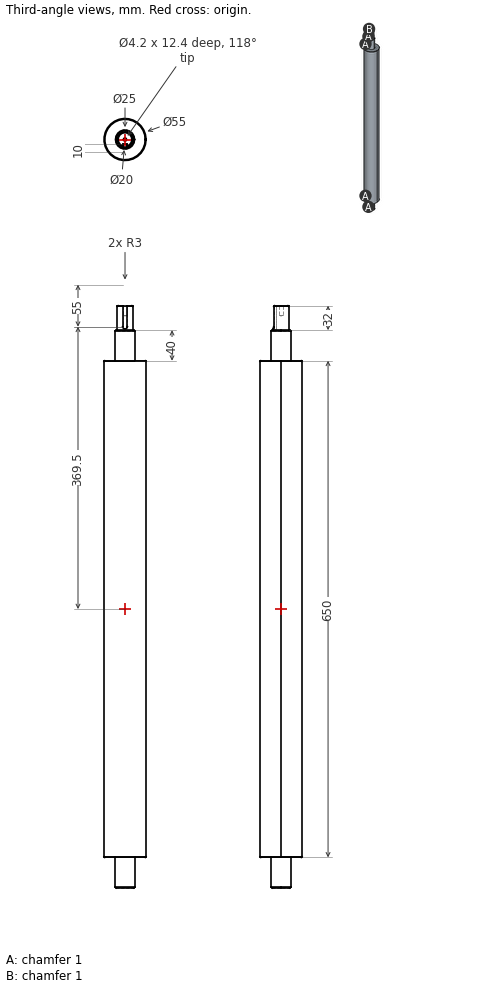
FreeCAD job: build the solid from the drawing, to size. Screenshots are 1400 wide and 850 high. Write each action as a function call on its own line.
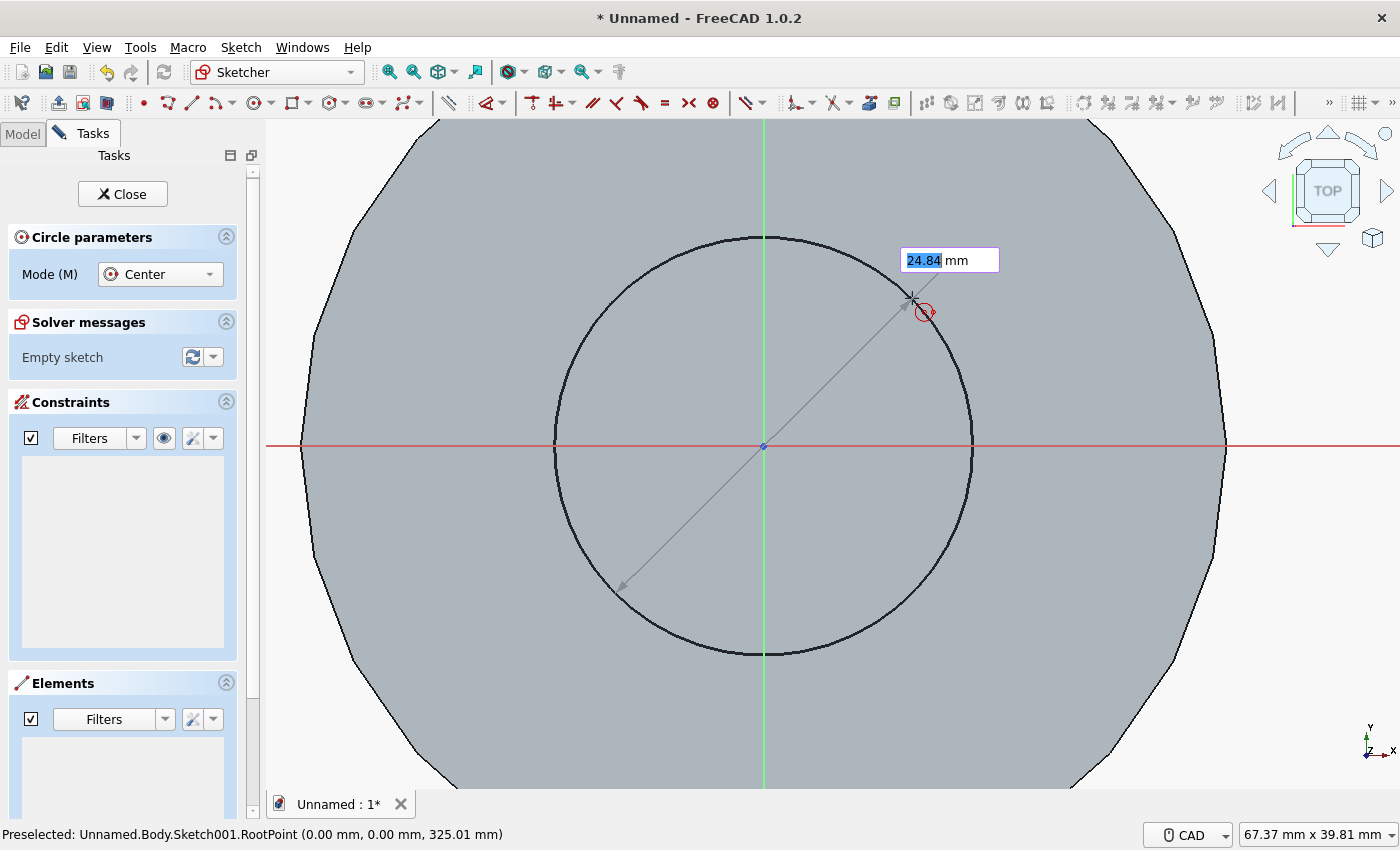
text(25)
key(Return)
key(Escape)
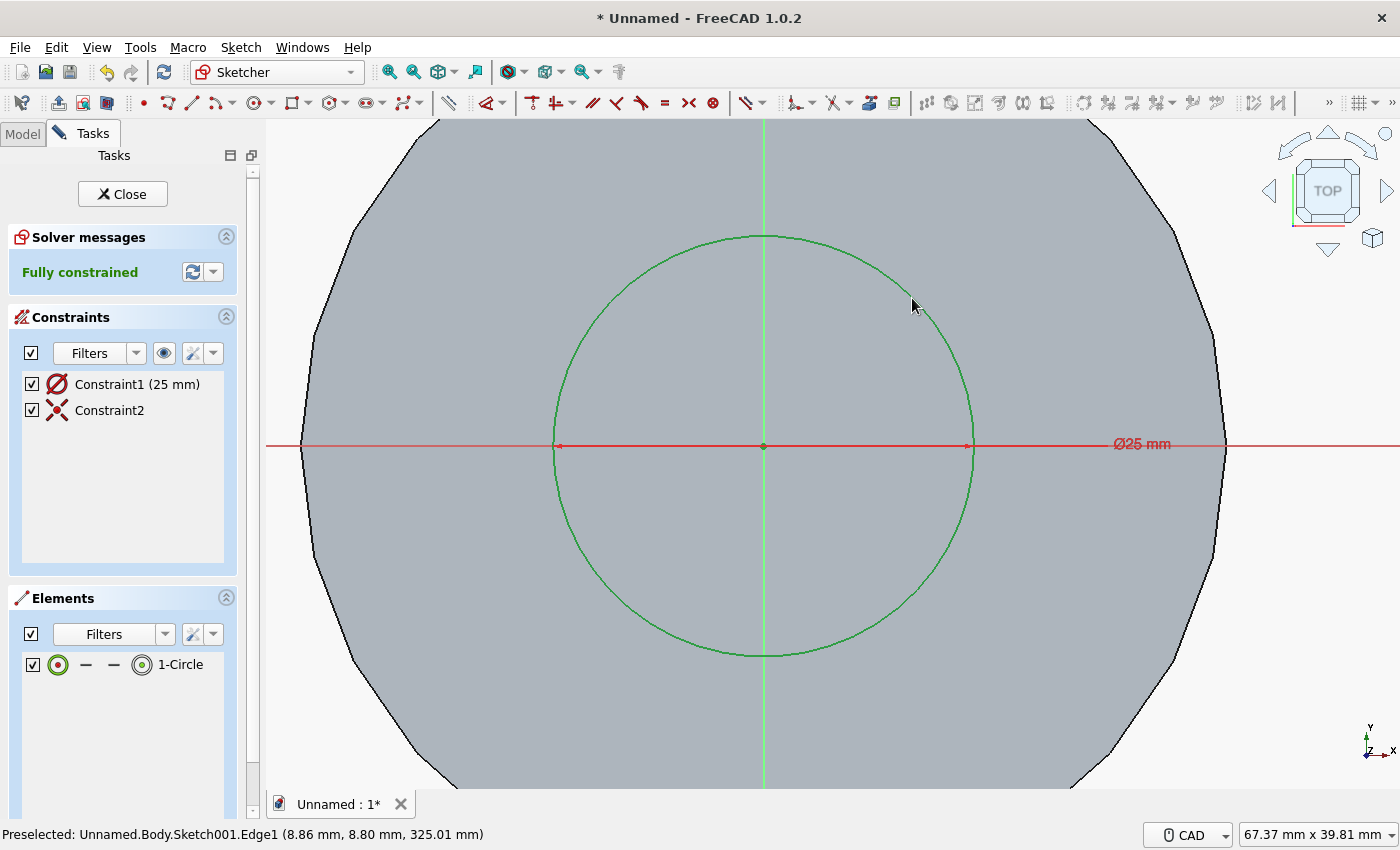
click(123, 194)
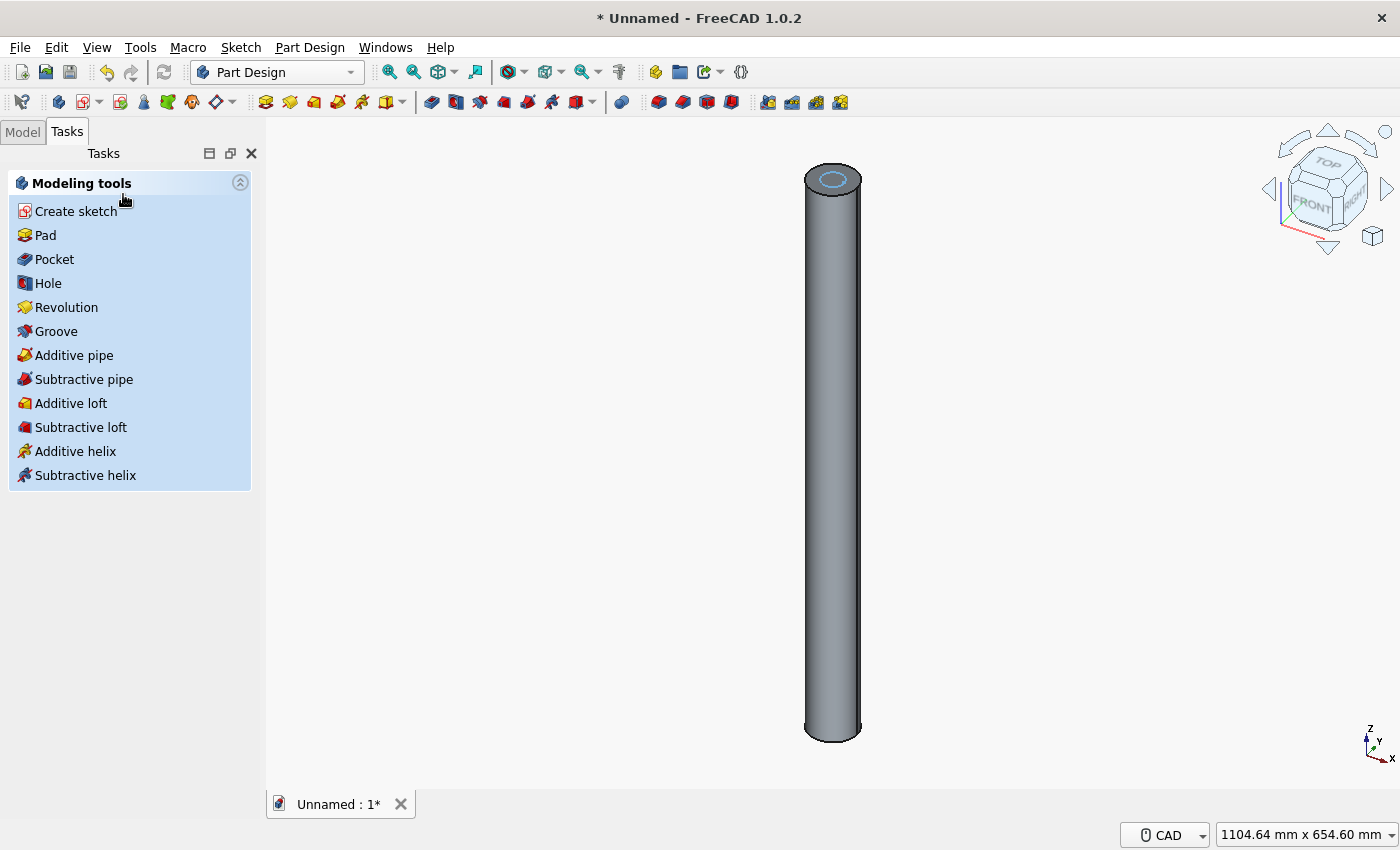
click(266, 102)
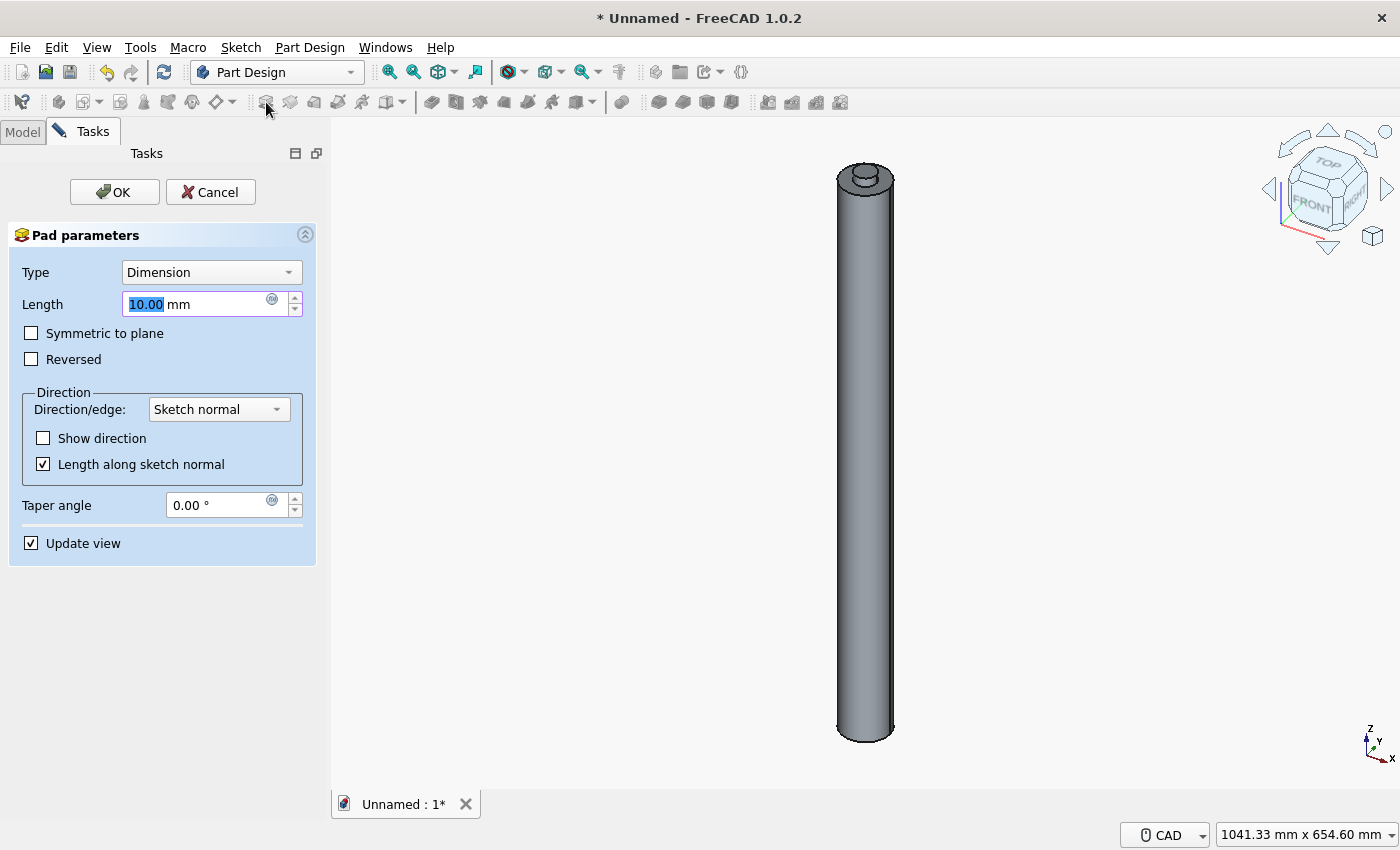
text(40)
key(Tab)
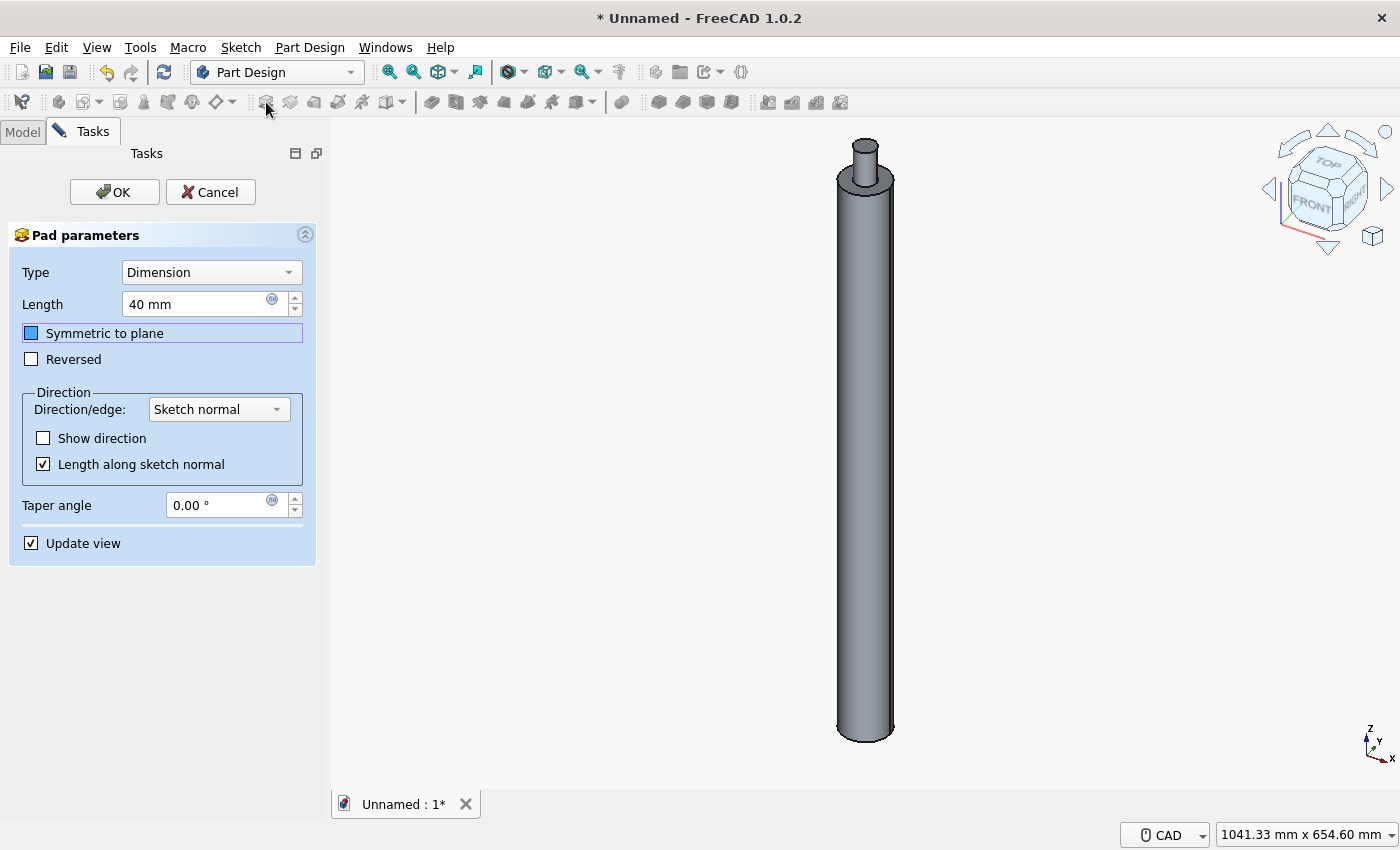
click(115, 192)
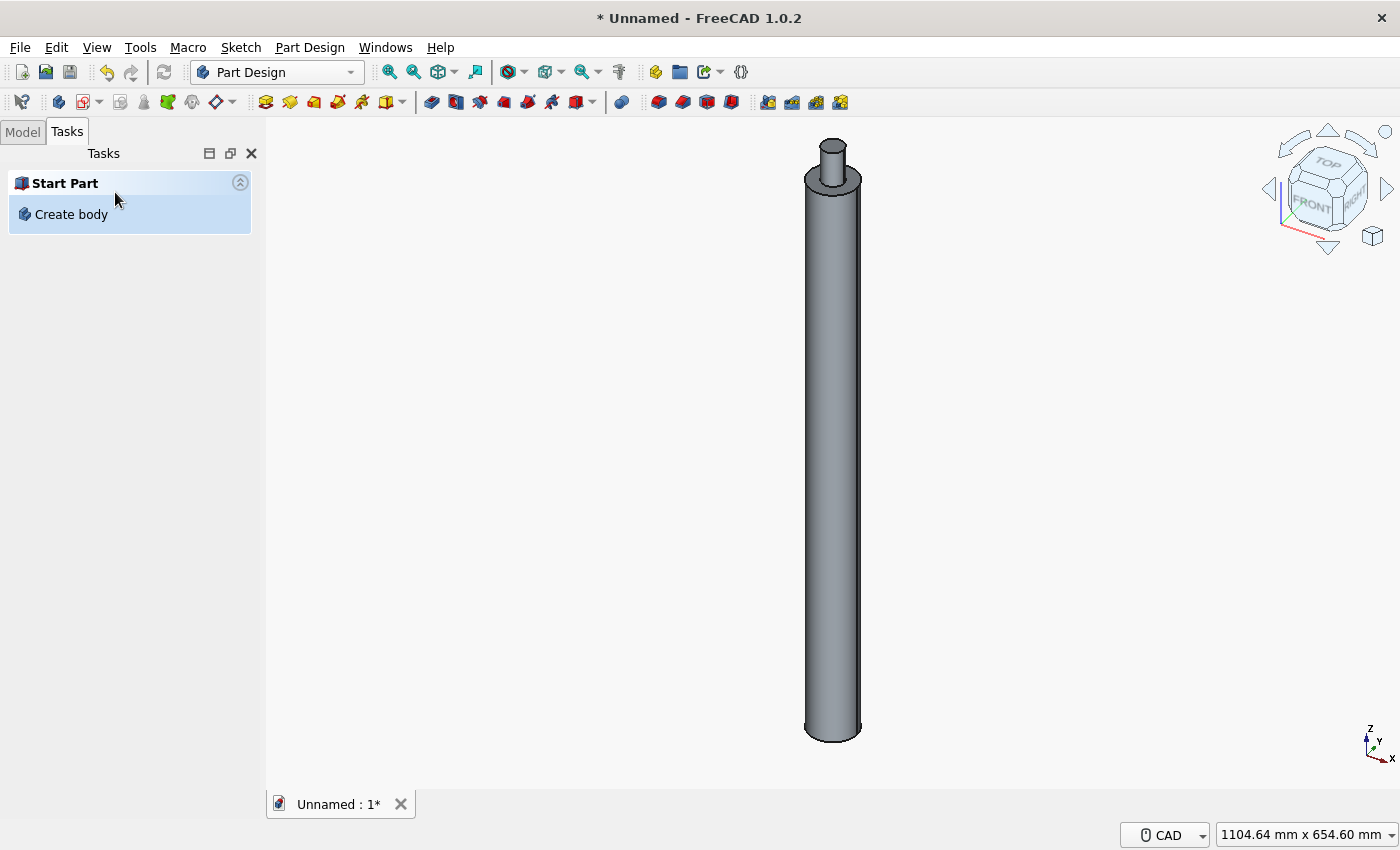
click(23, 131)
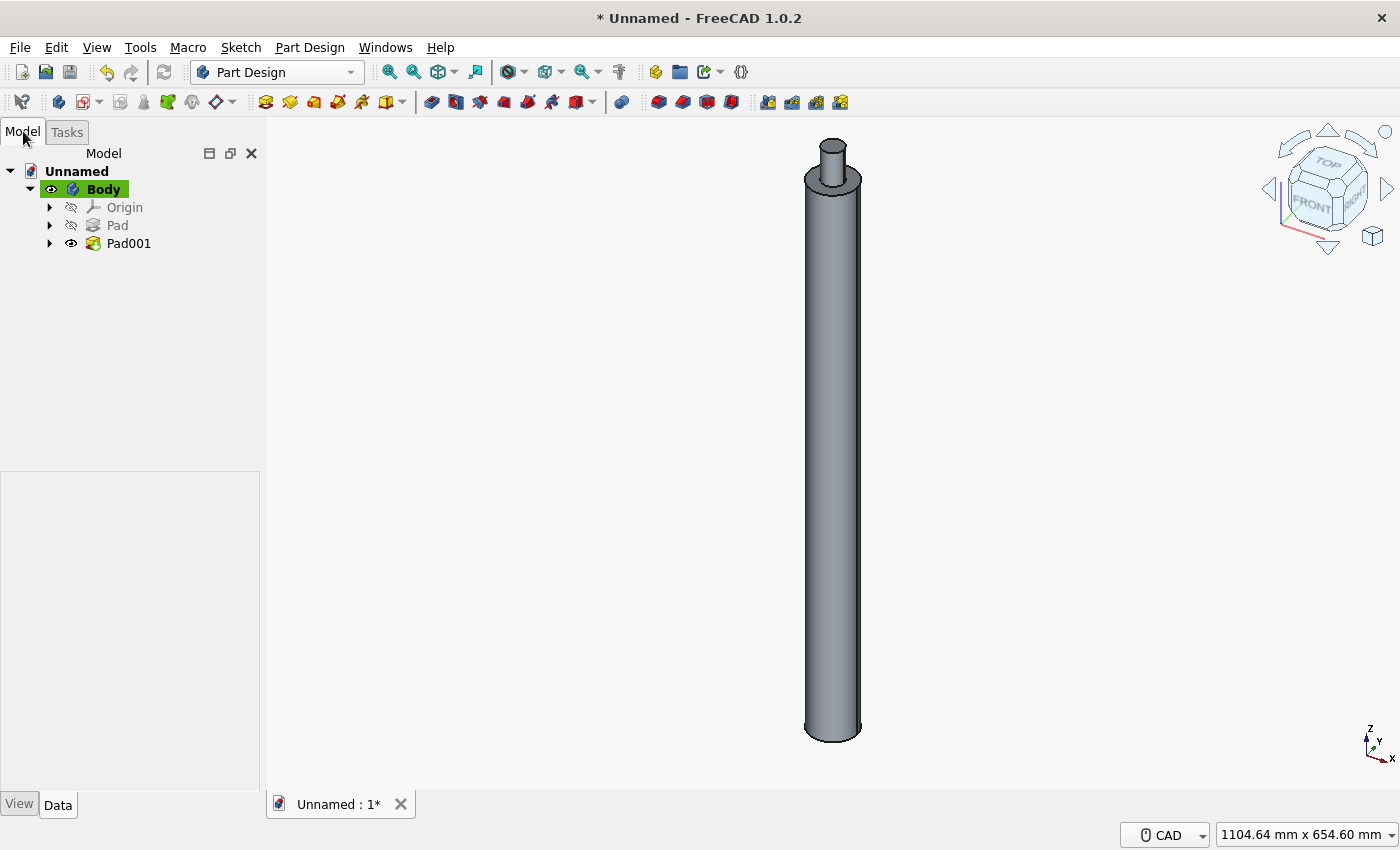
click(116, 243)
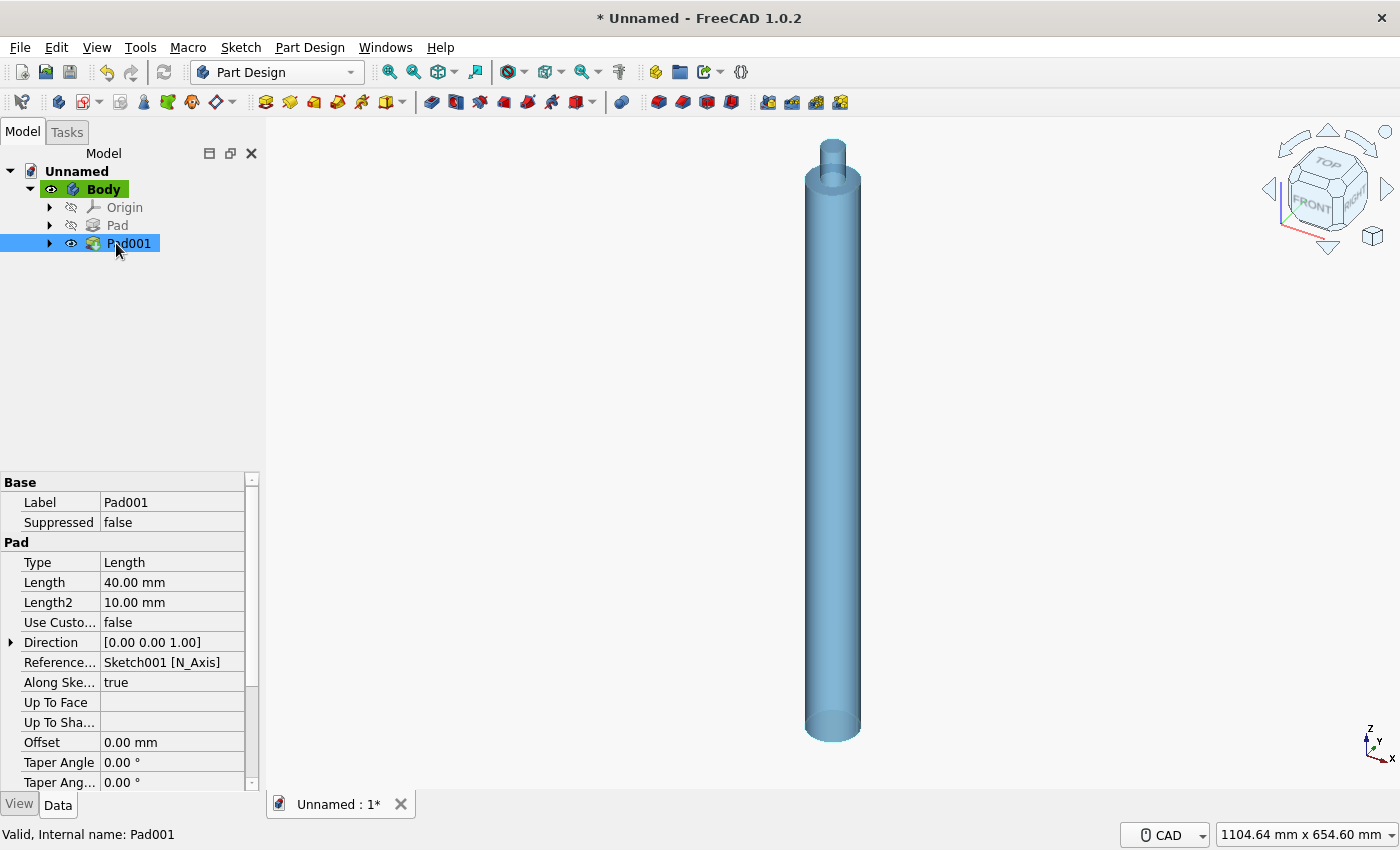
click(768, 102)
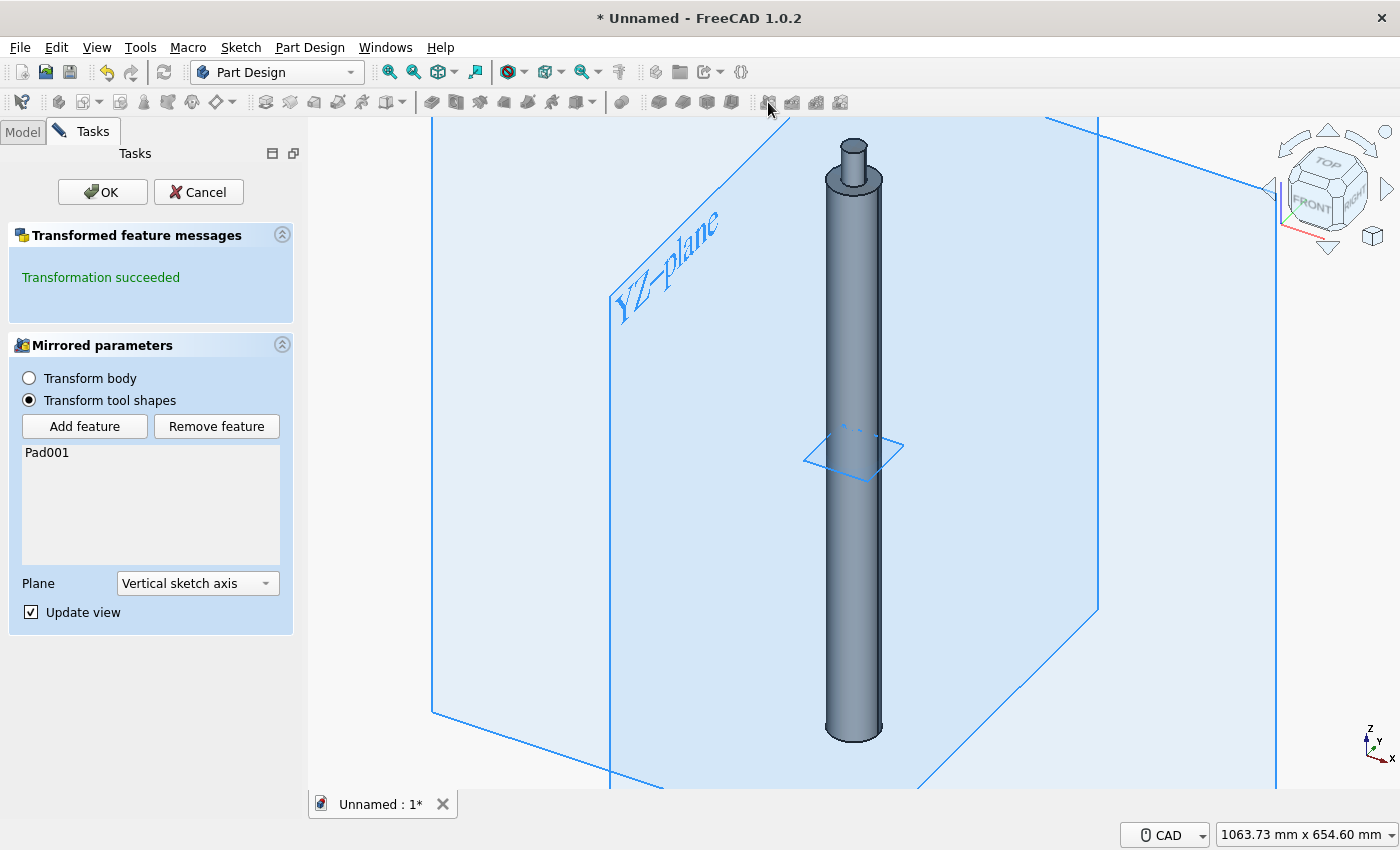
click(198, 584)